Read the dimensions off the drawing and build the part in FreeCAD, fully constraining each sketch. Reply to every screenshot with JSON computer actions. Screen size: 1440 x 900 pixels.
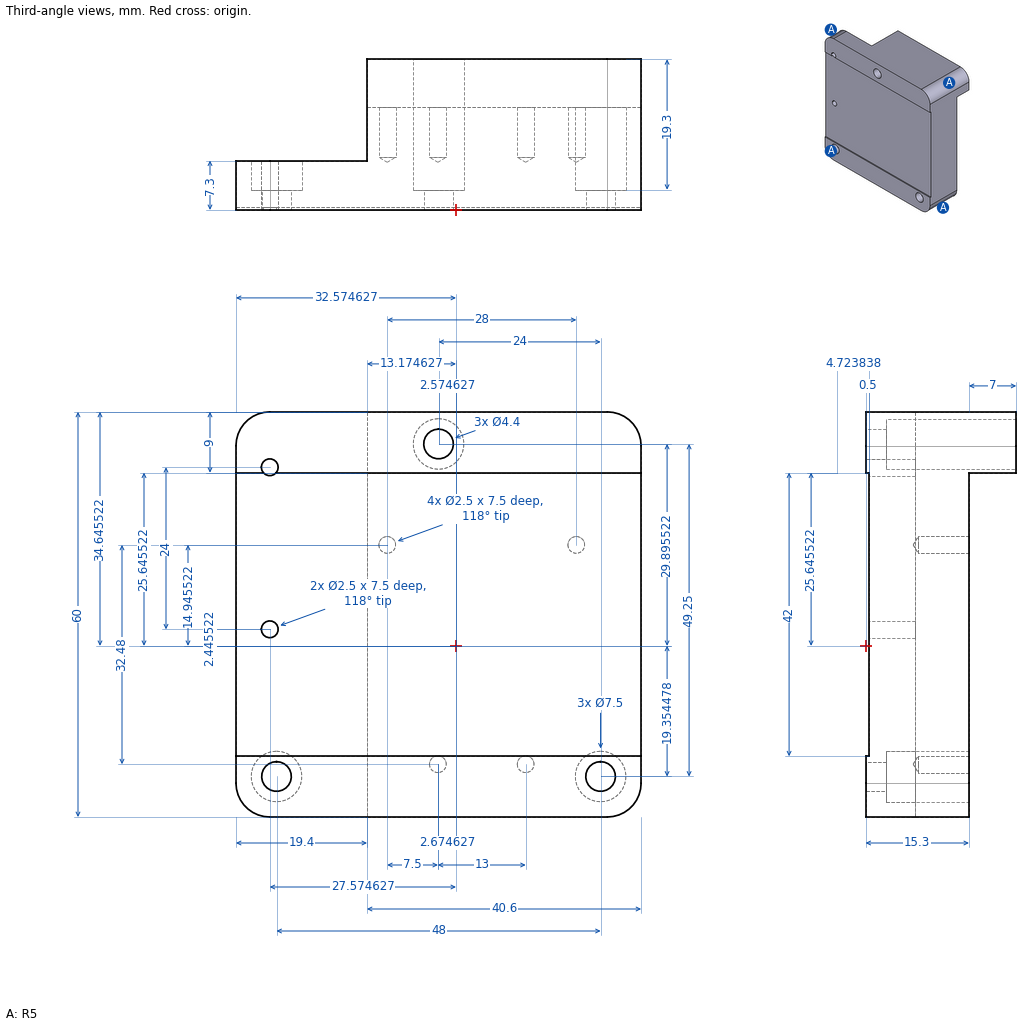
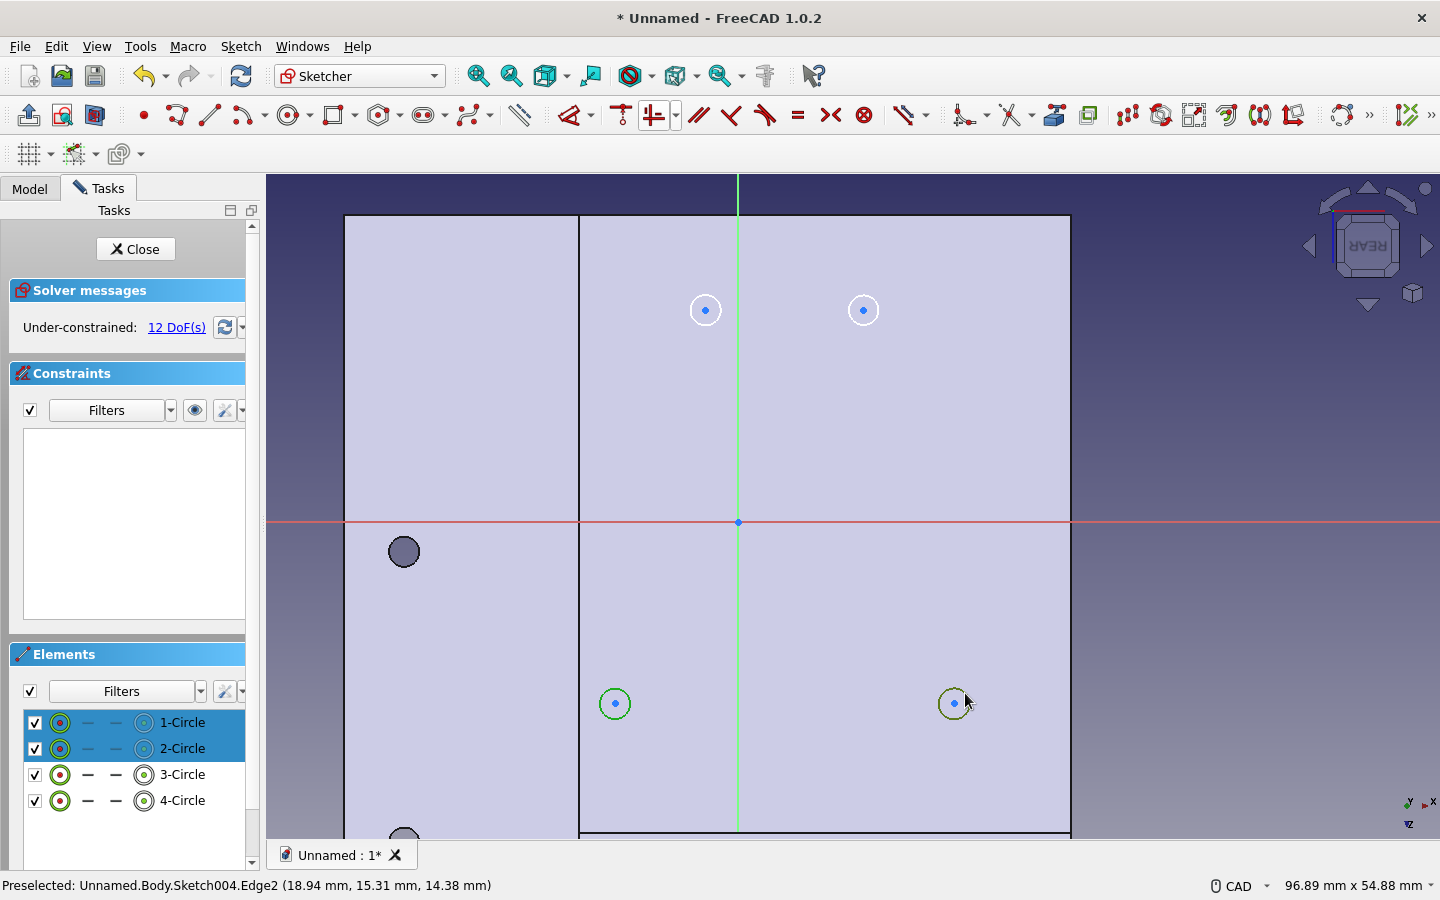
{"action": "left_click", "coordinate": [716, 299]}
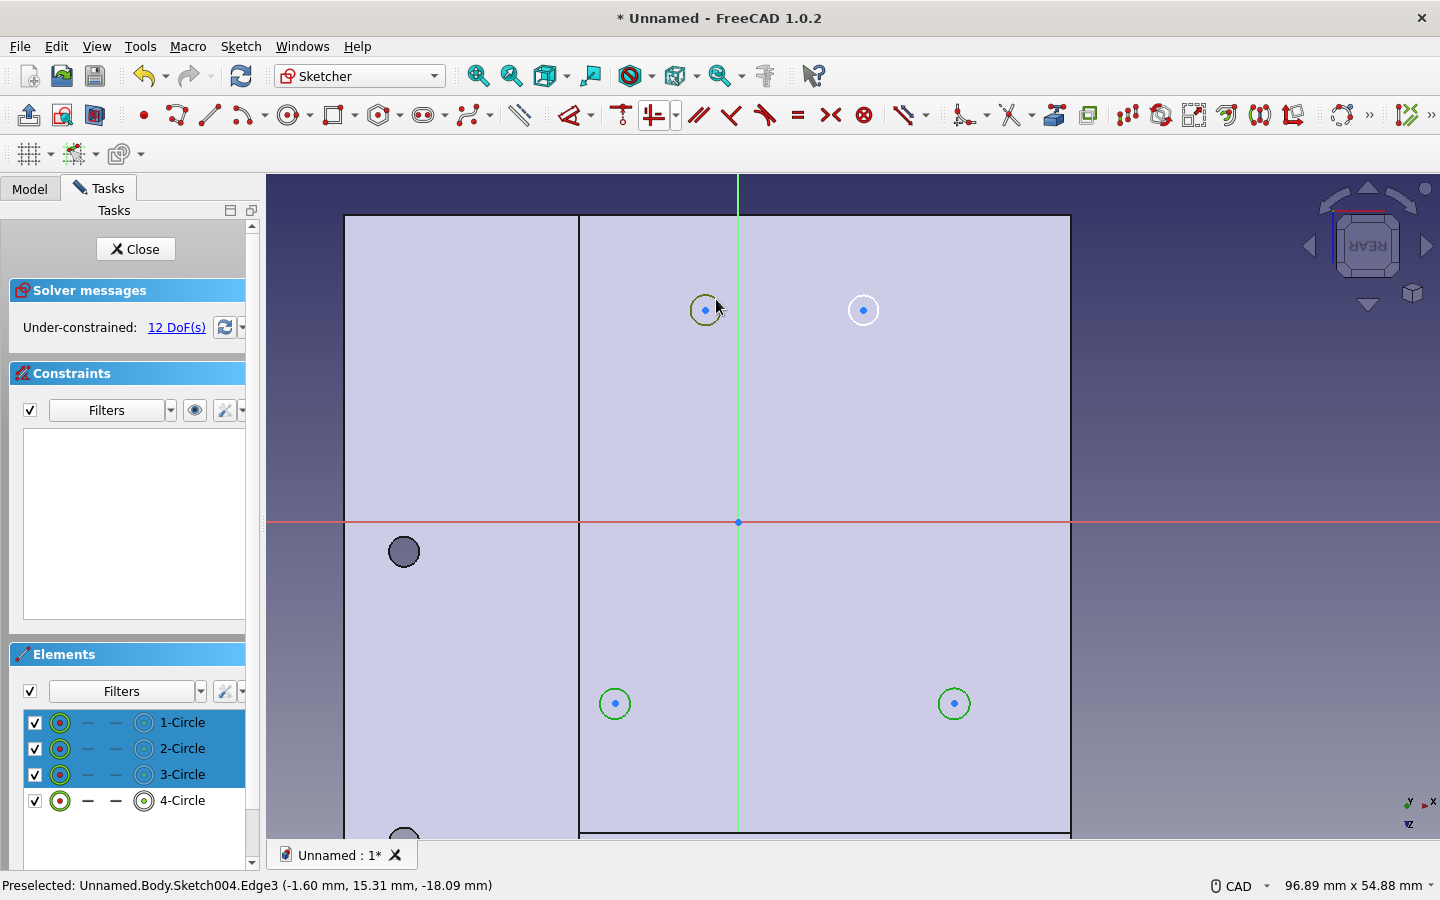
{"action": "left_click", "coordinate": [874, 300]}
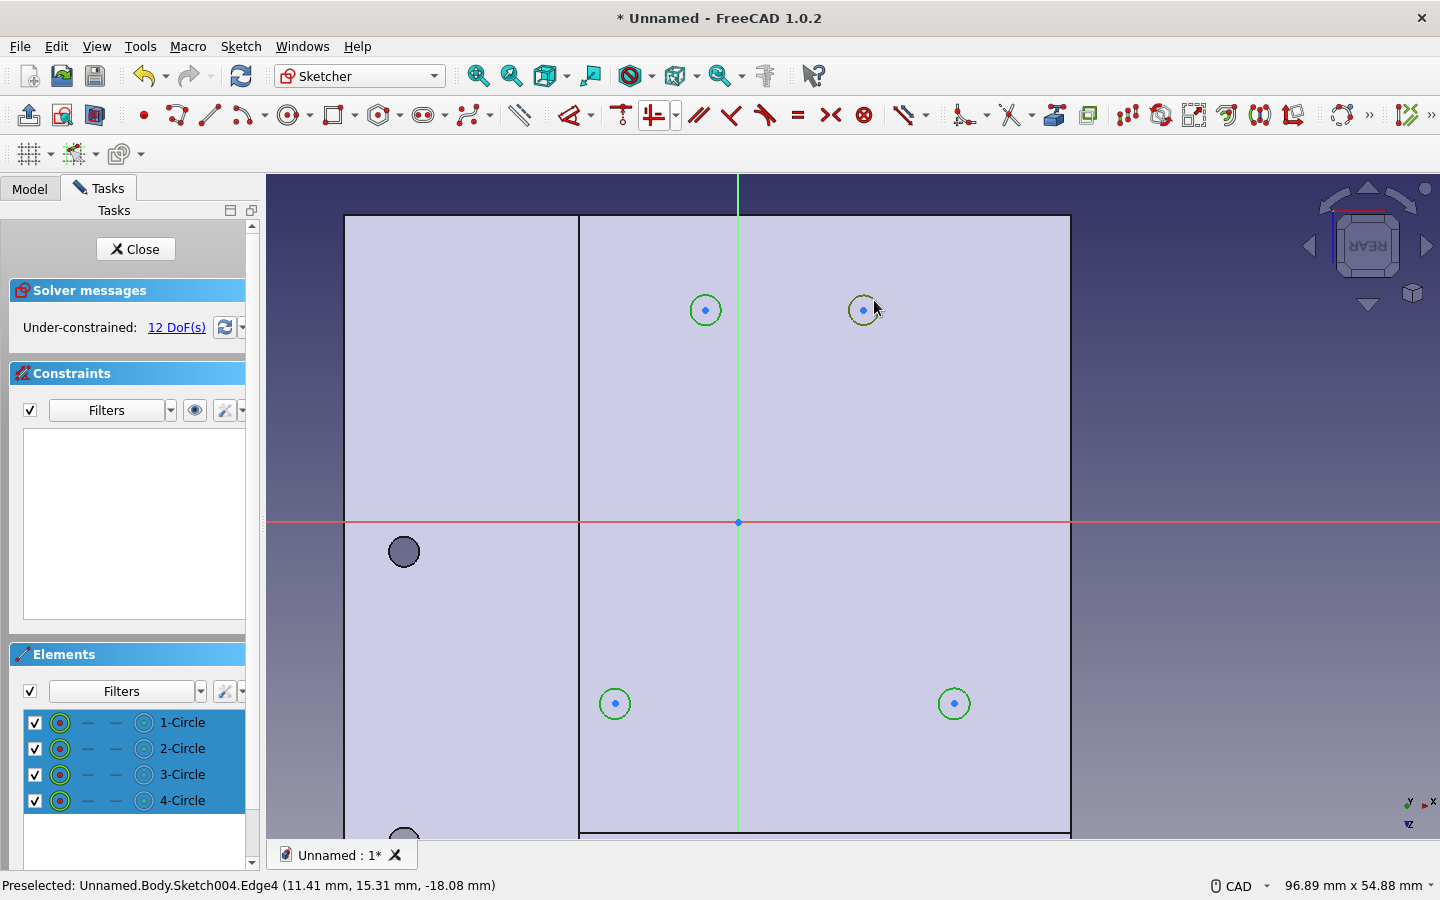
{"action": "key", "text": "e"}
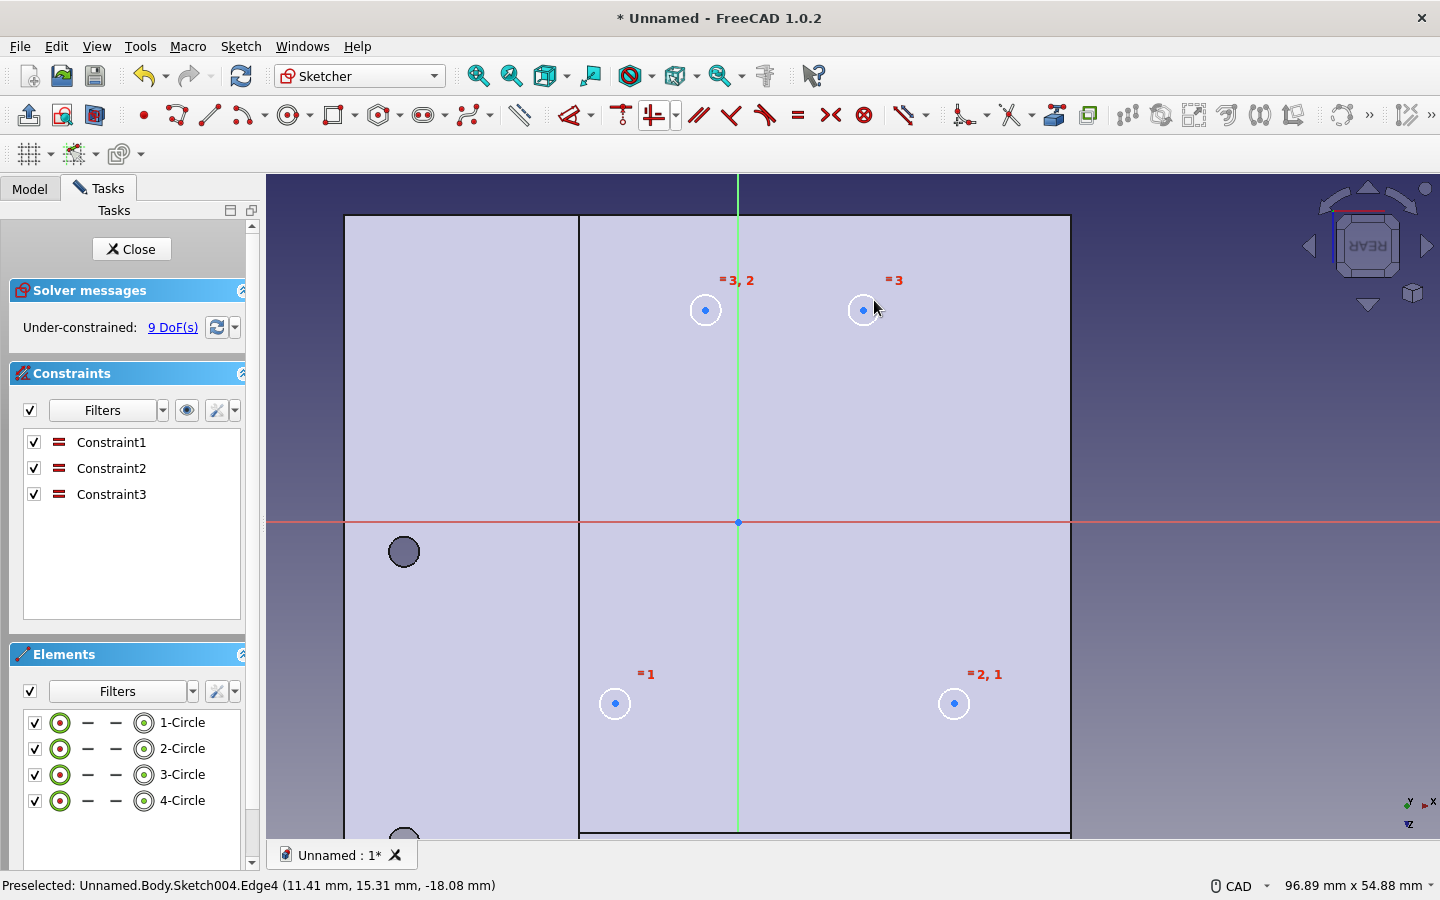
{"action": "left_click", "coordinate": [615, 704]}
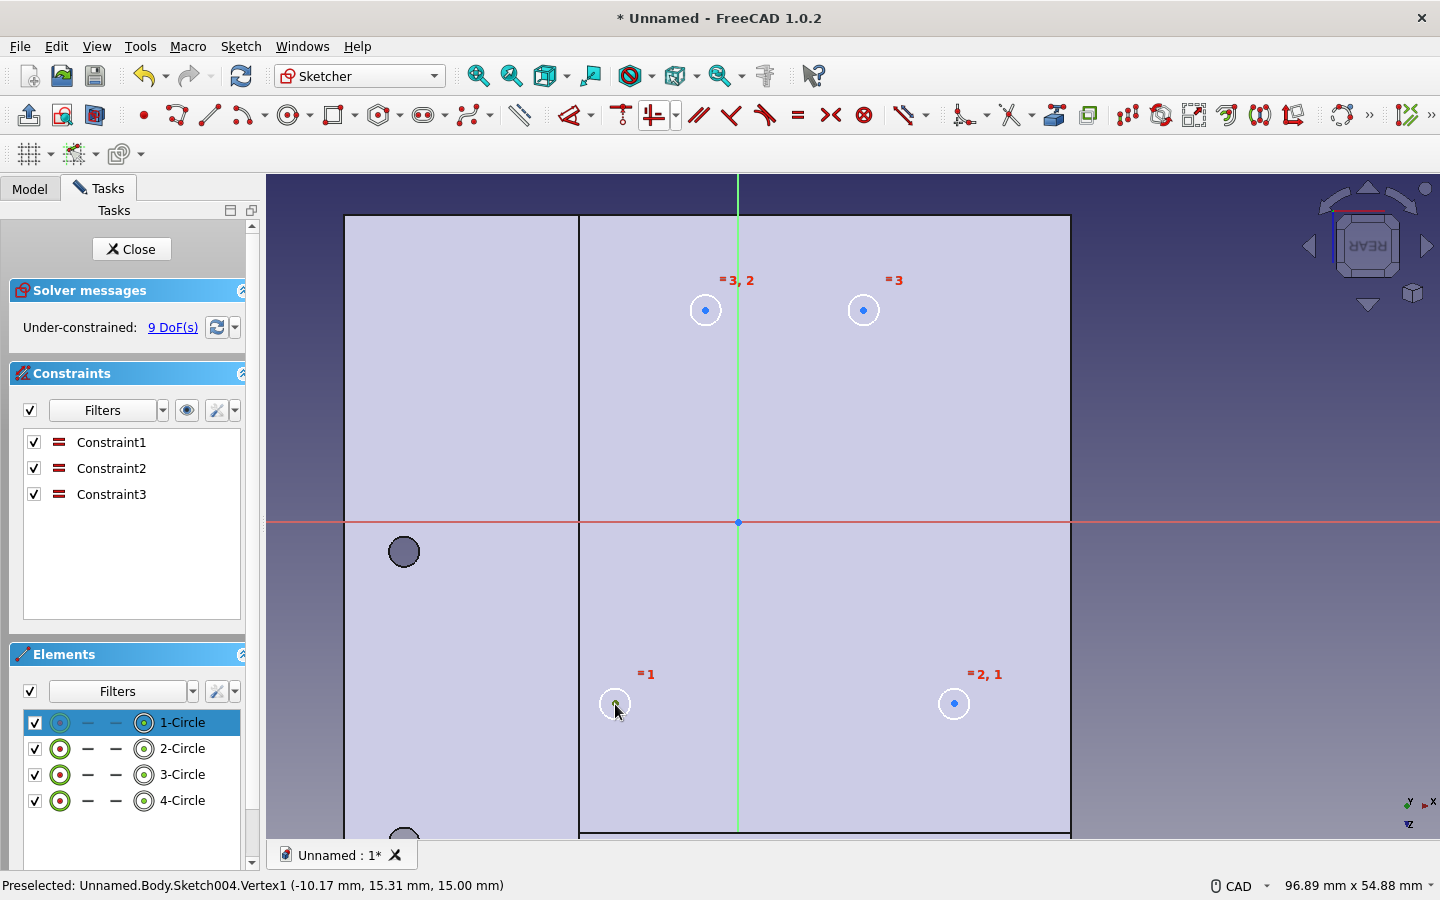
{"action": "left_click", "coordinate": [954, 704]}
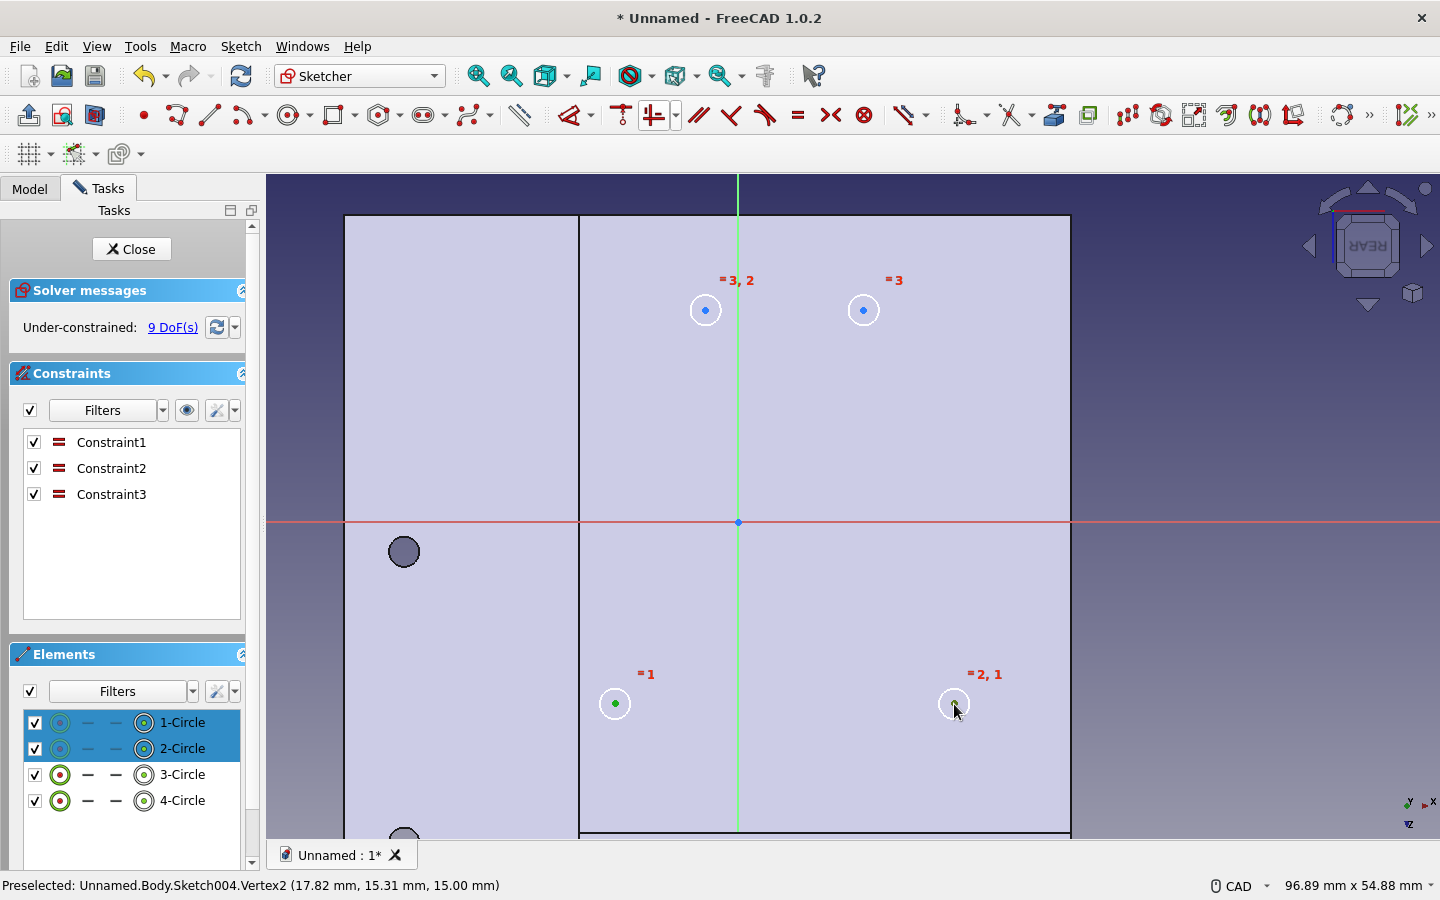
{"action": "key", "text": "h"}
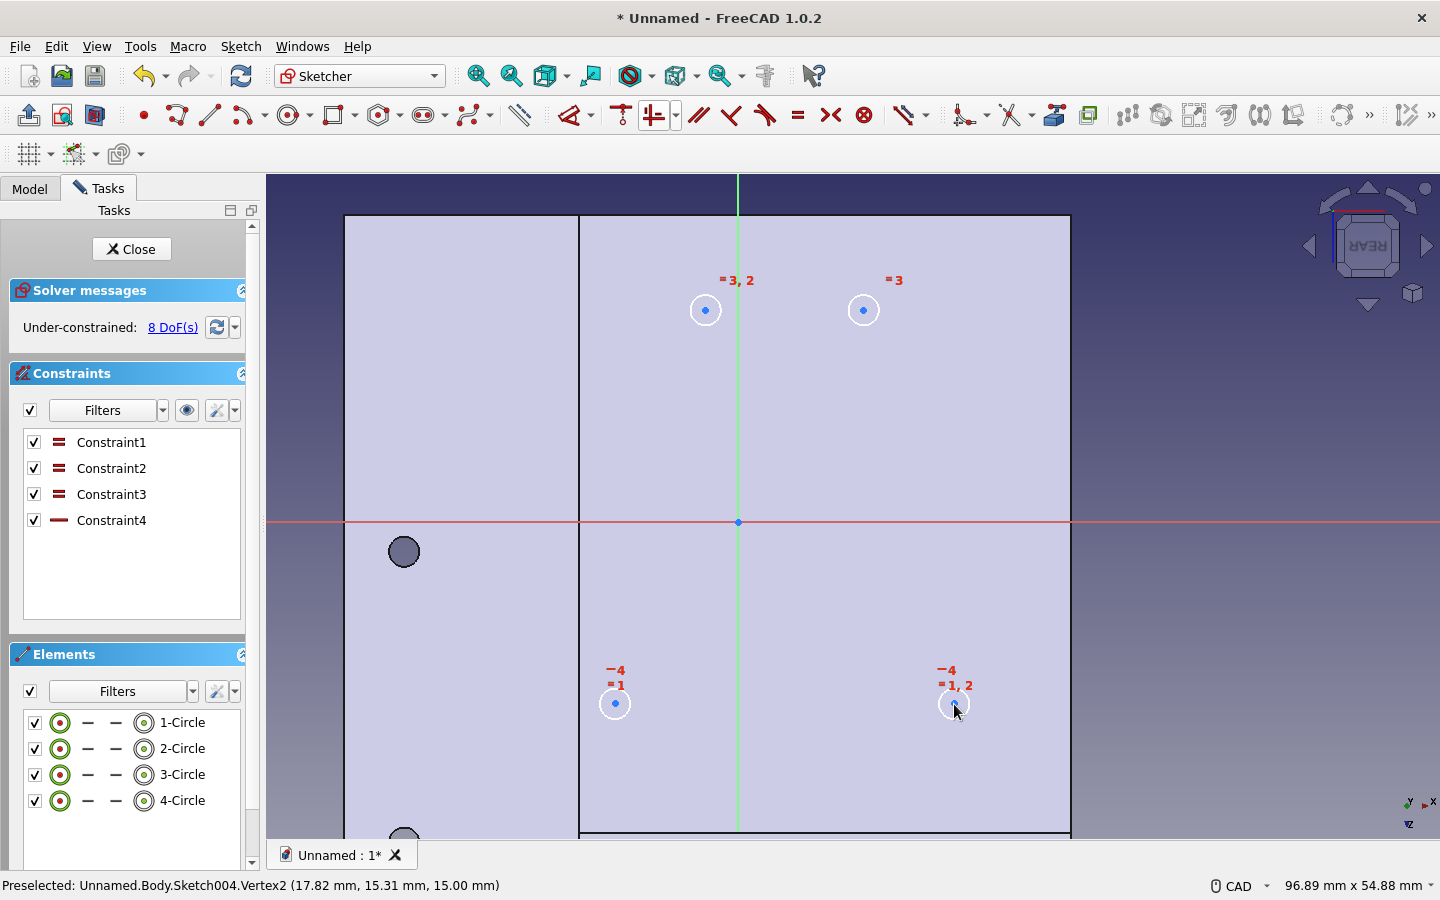
{"action": "left_click", "coordinate": [706, 310]}